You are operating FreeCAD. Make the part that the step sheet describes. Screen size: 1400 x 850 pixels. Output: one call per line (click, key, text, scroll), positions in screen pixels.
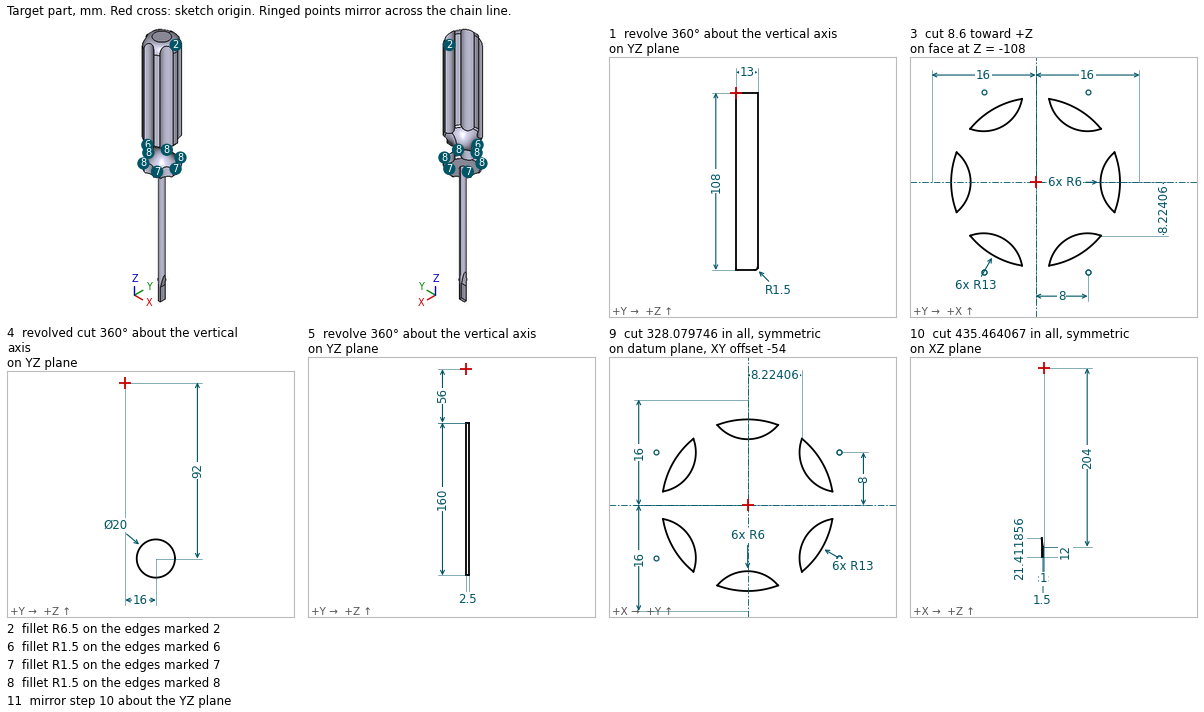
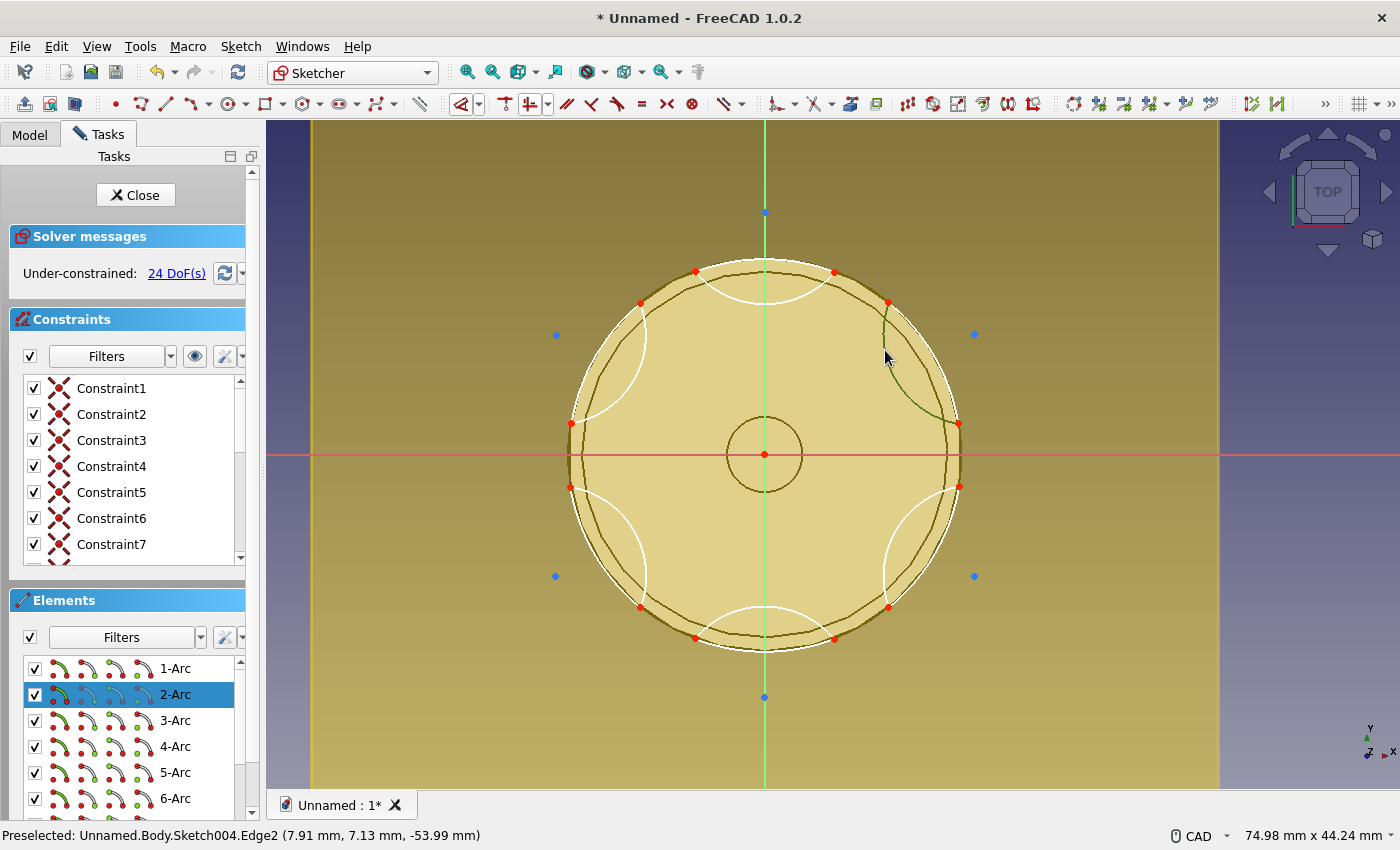
click(916, 507)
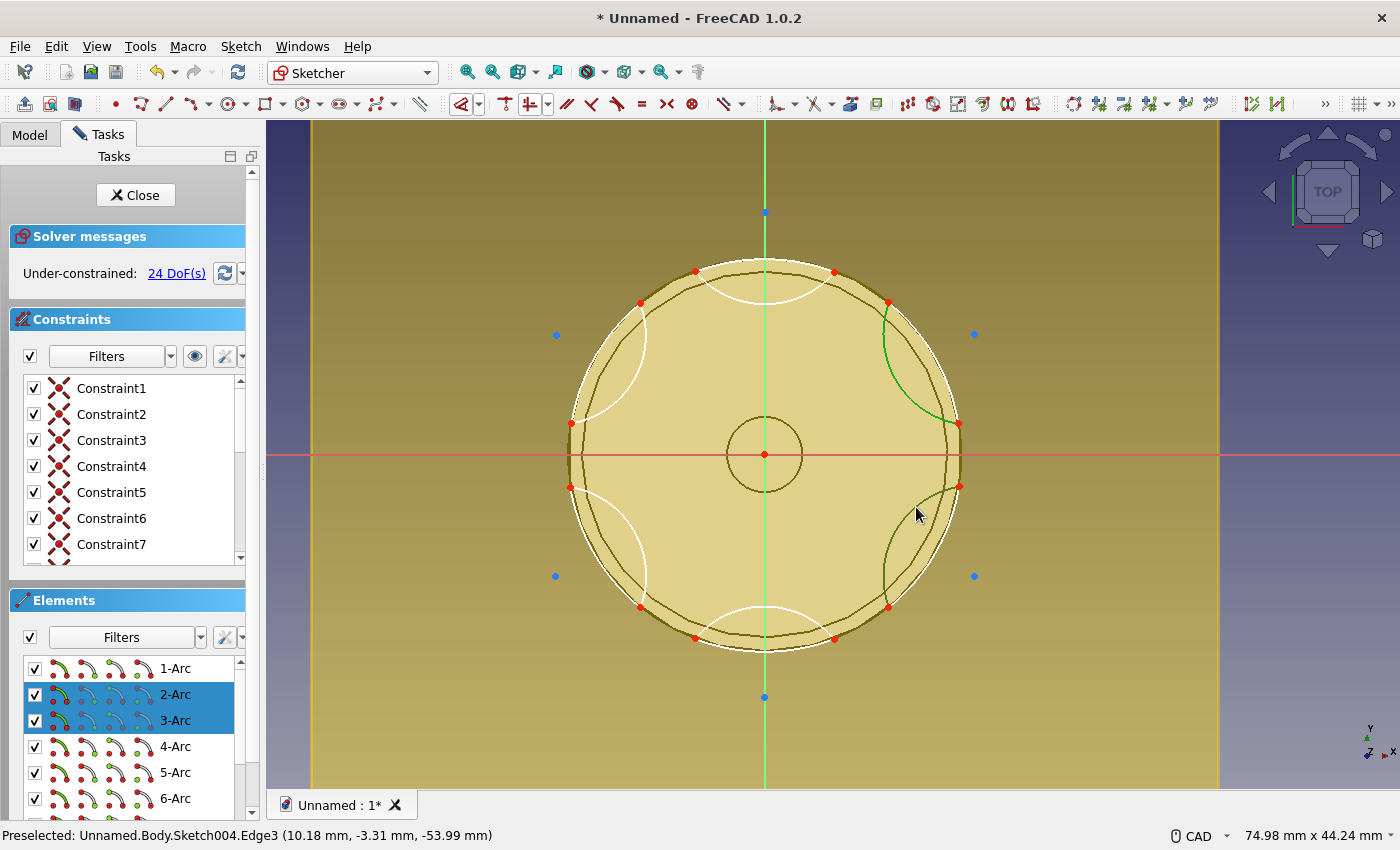
click(796, 612)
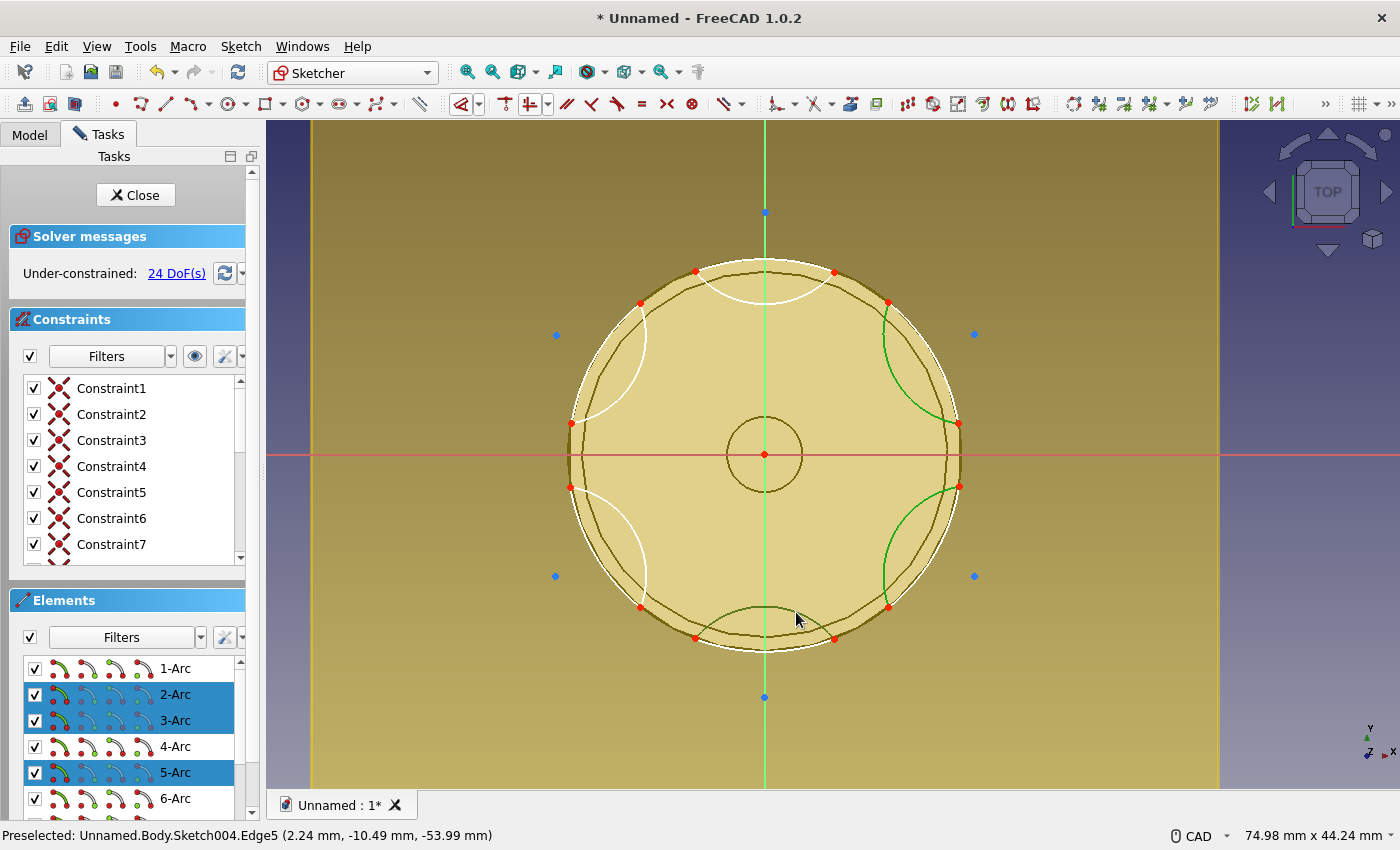
click(645, 561)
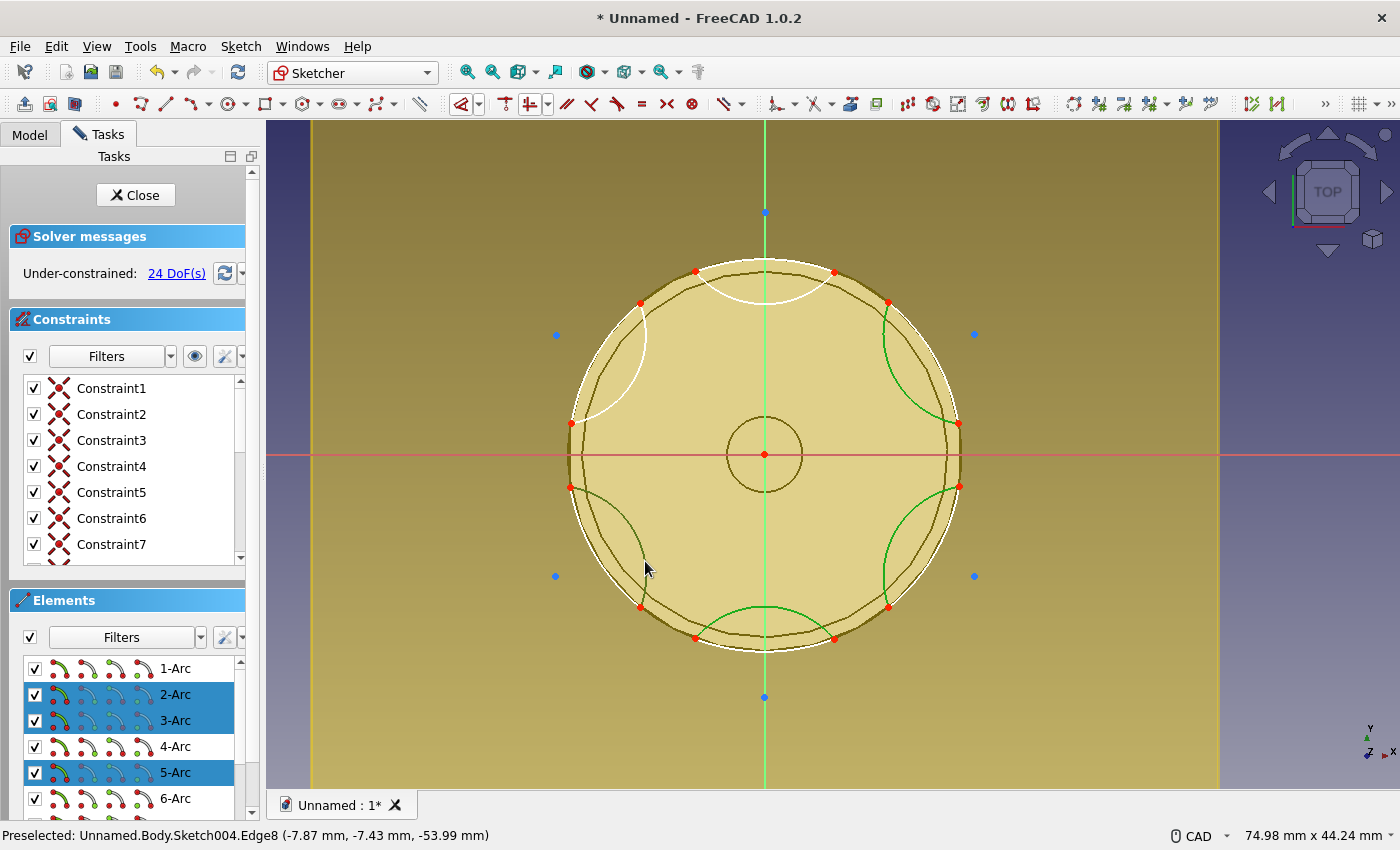
click(614, 404)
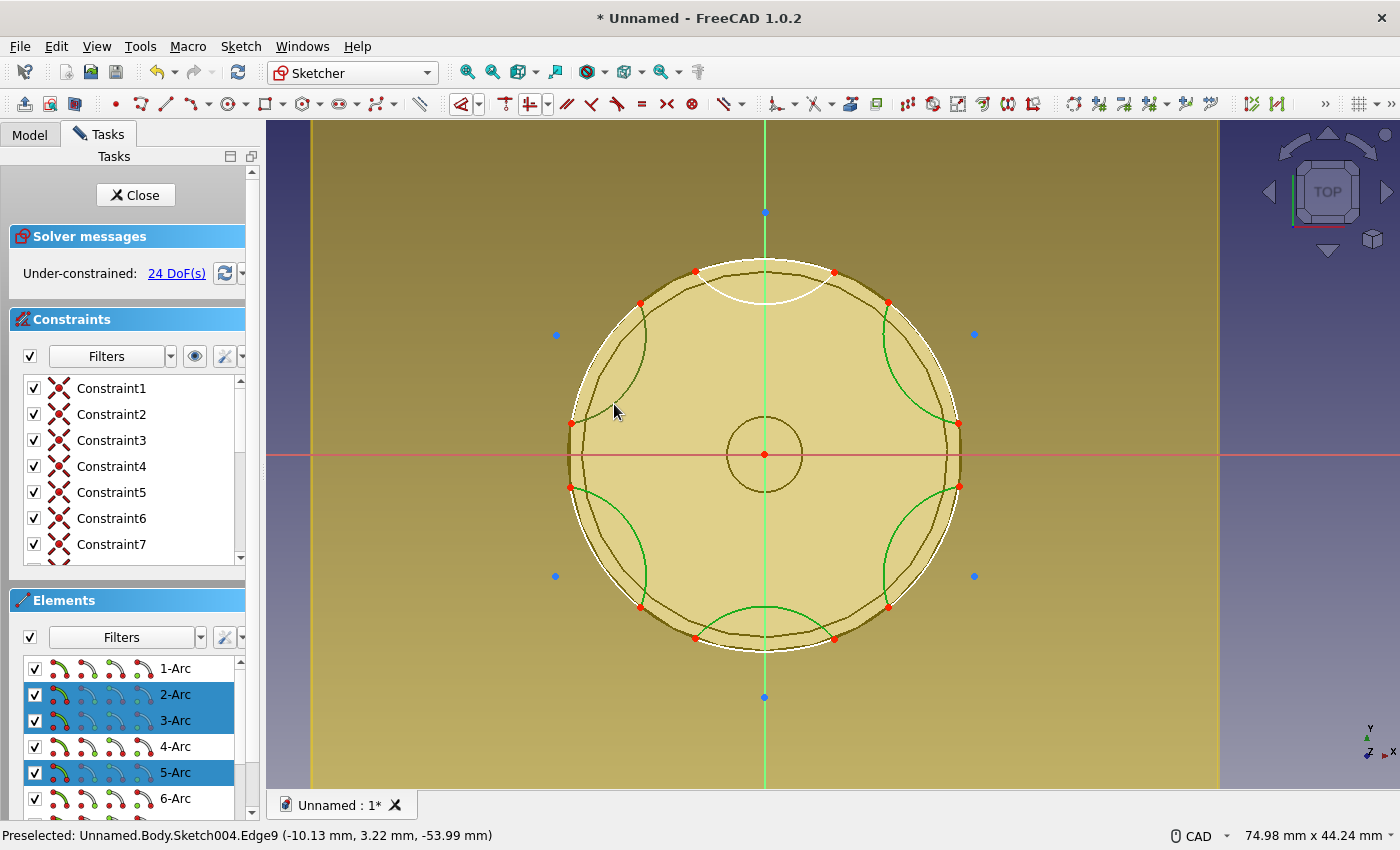
click(734, 299)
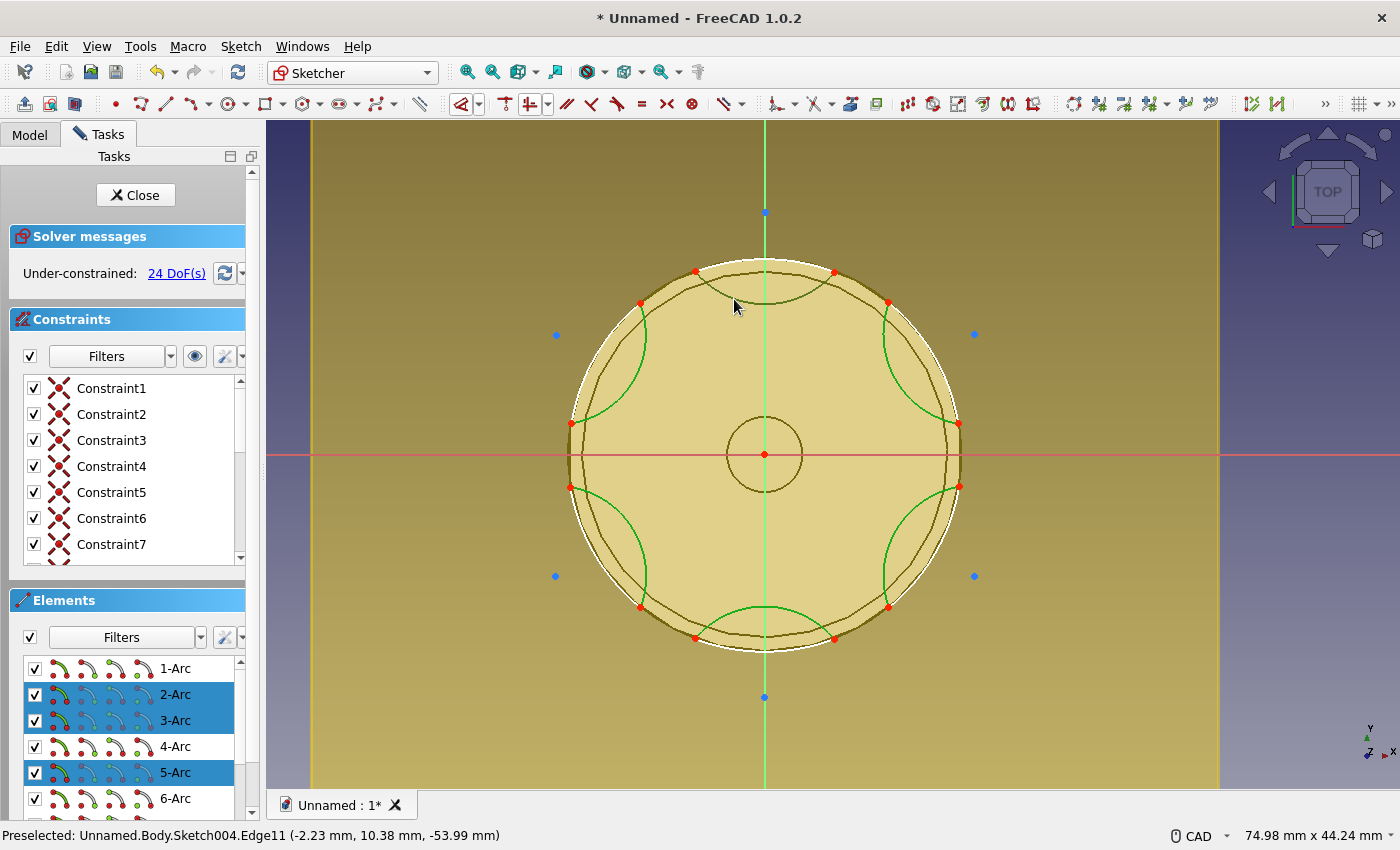
key(e)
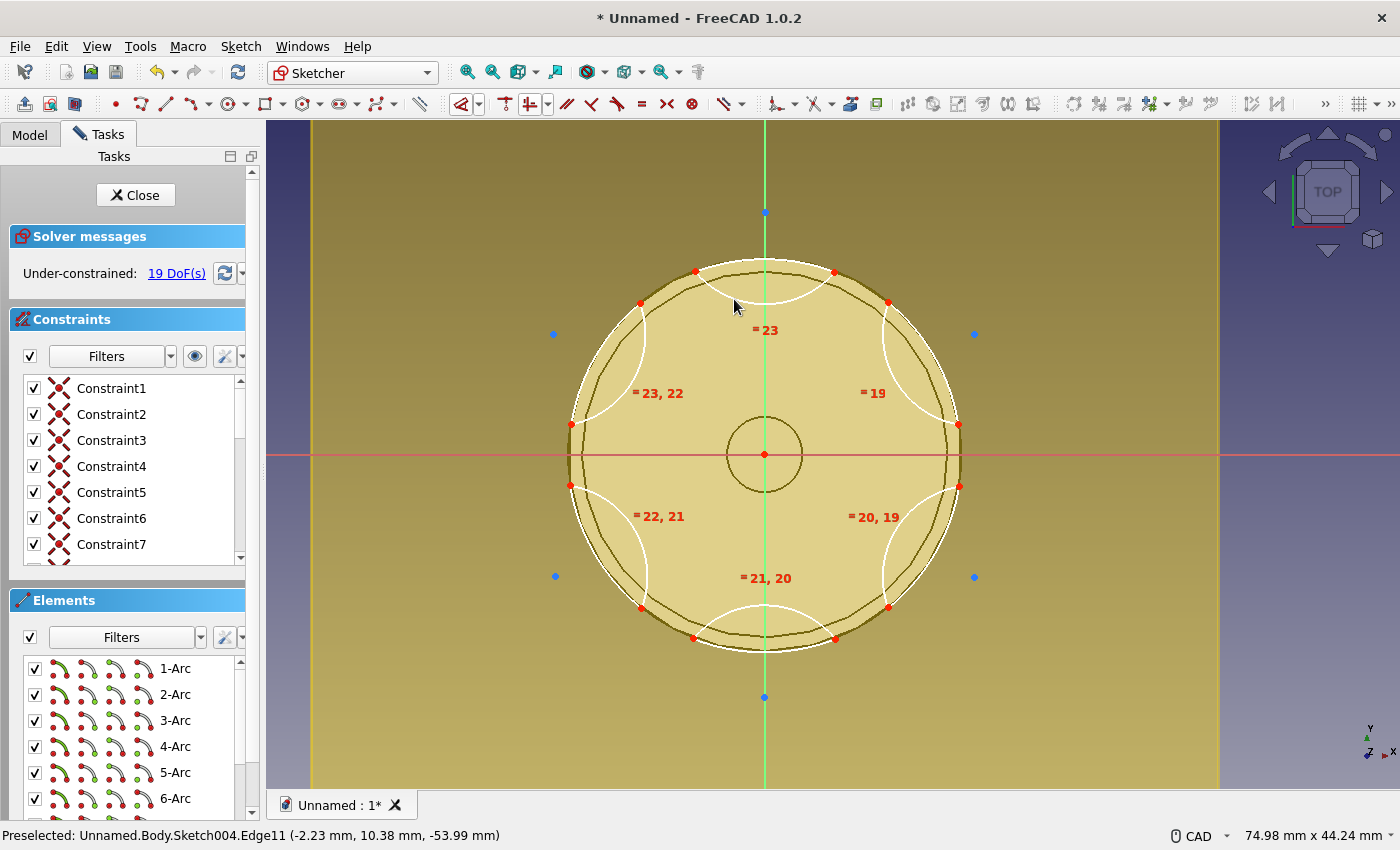
click(947, 383)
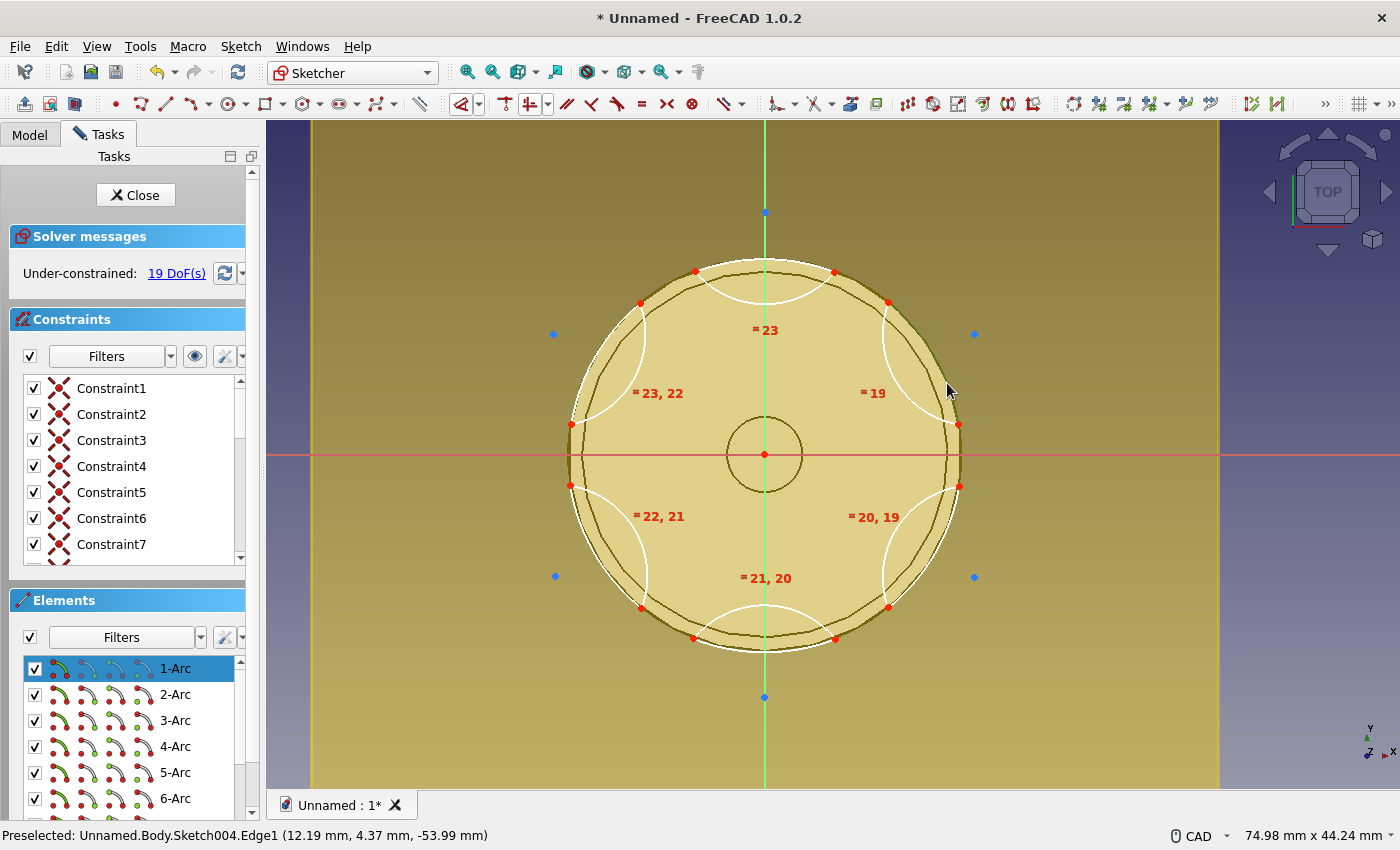
click(919, 578)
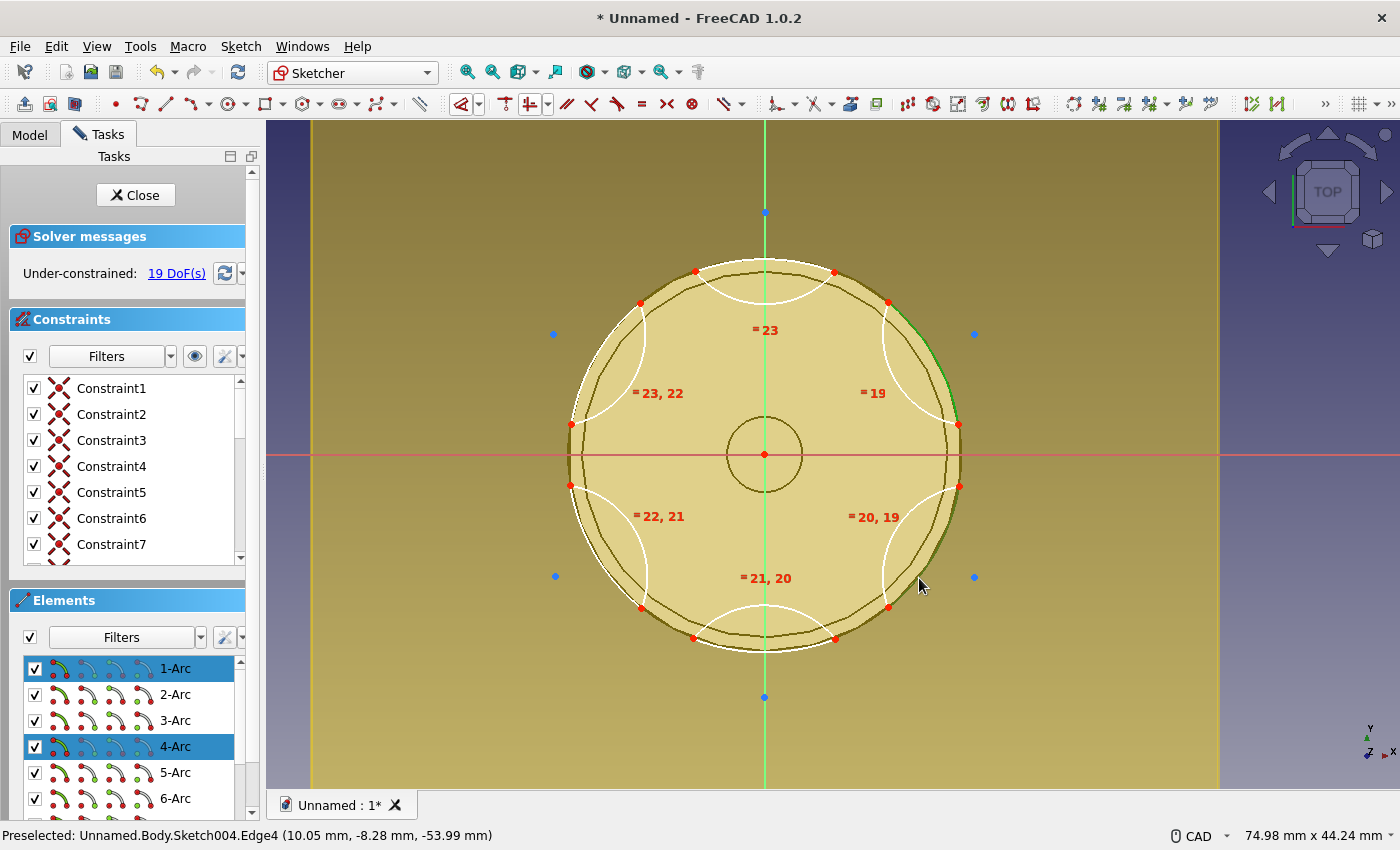
click(736, 650)